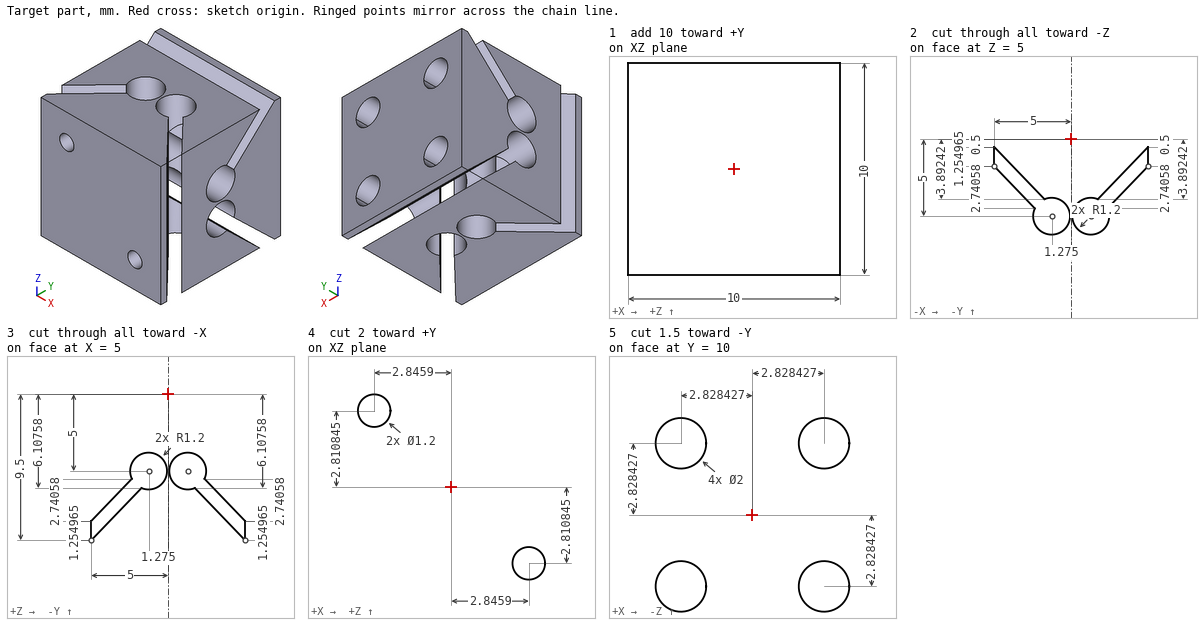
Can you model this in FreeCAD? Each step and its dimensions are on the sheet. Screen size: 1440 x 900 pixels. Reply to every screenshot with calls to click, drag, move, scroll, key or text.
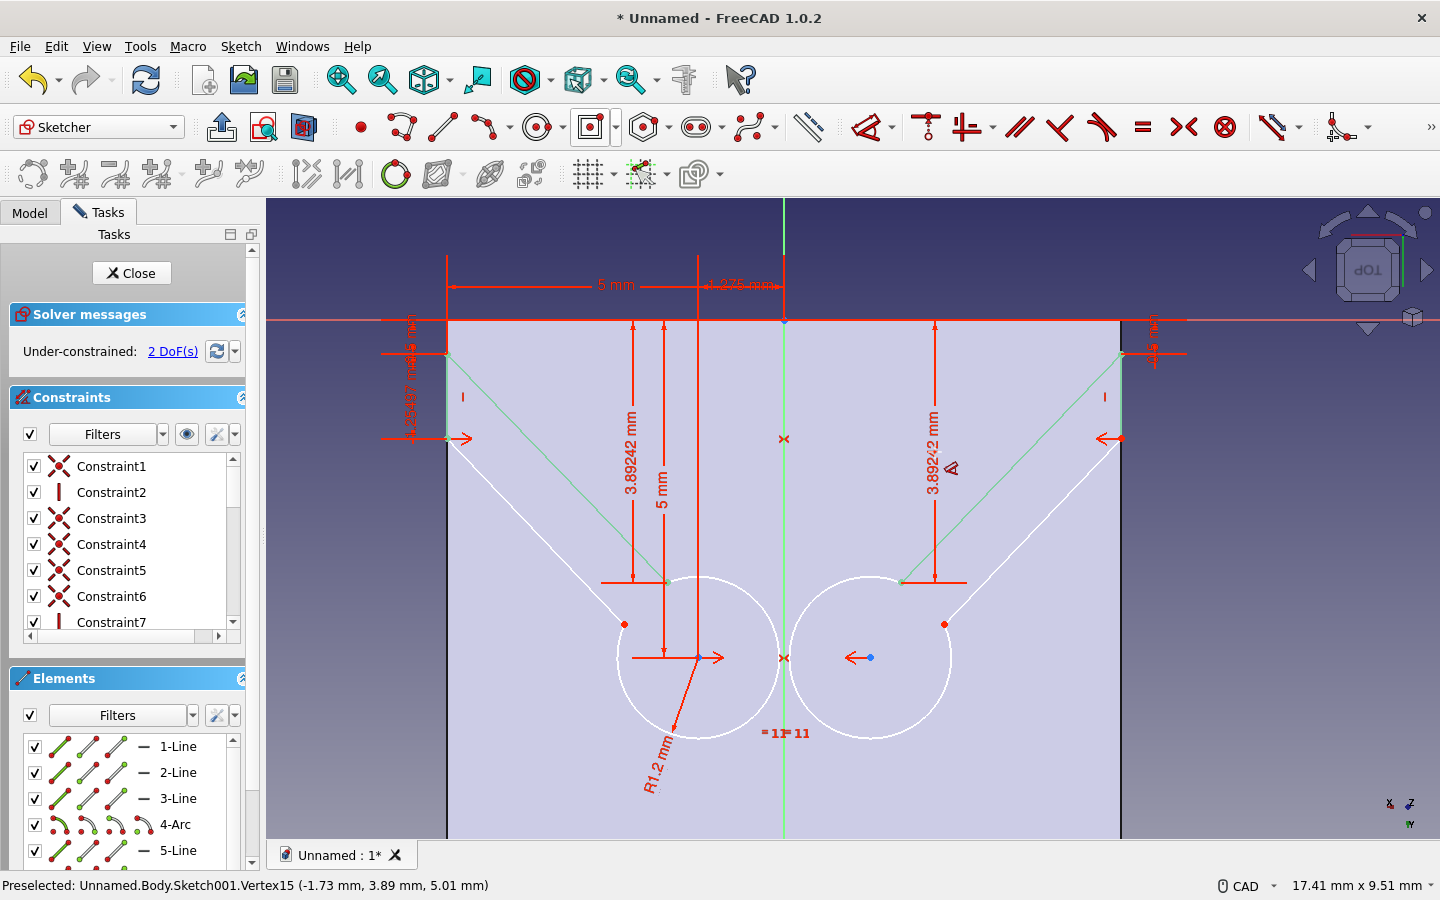
click(500, 495)
click(413, 532)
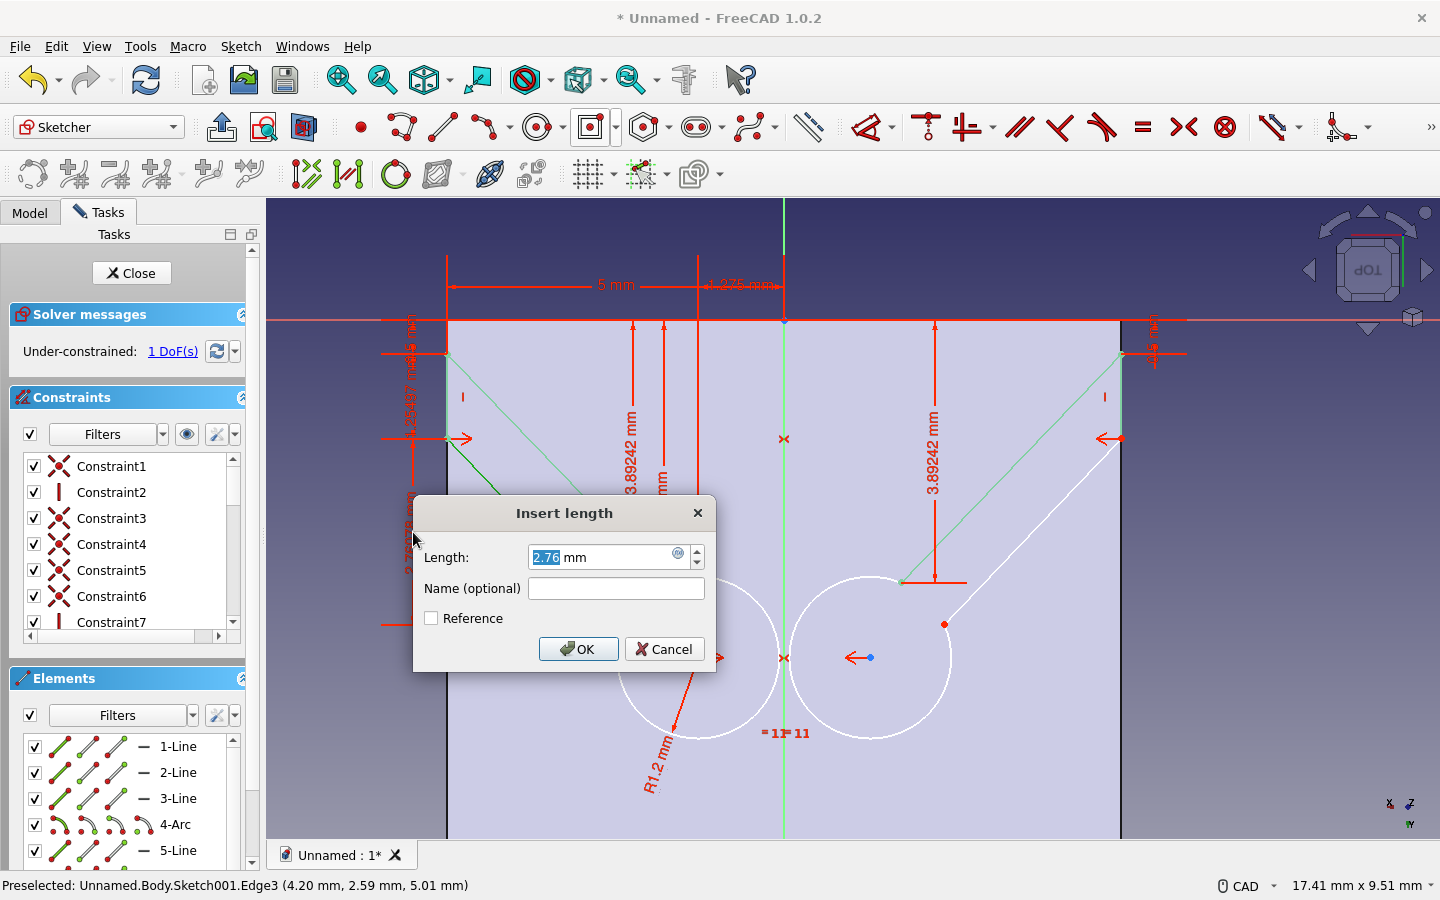
text(2.74058)
key(Return)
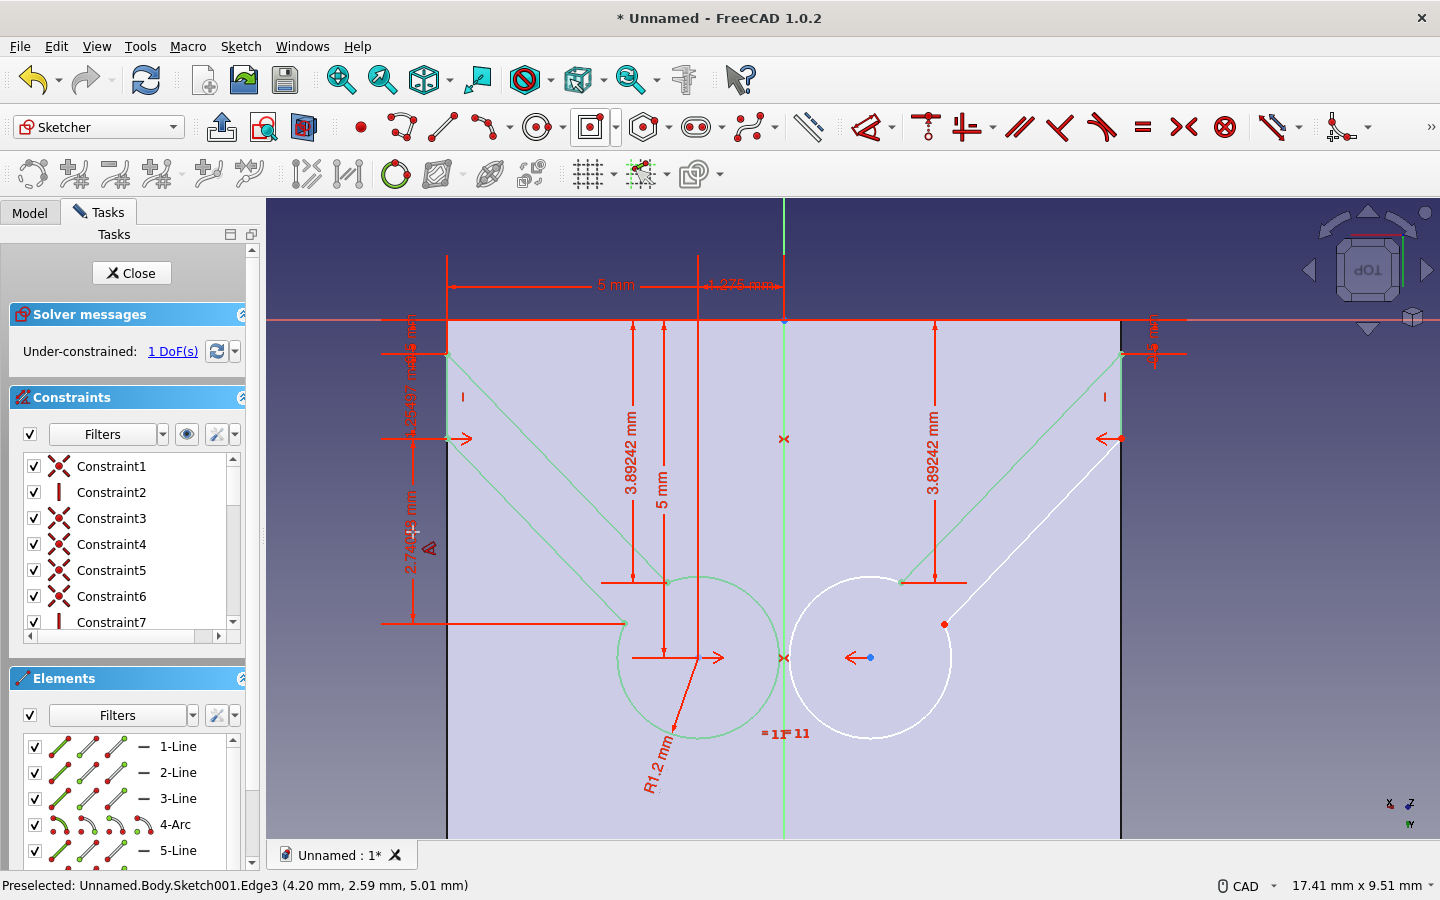
click(997, 569)
click(1155, 532)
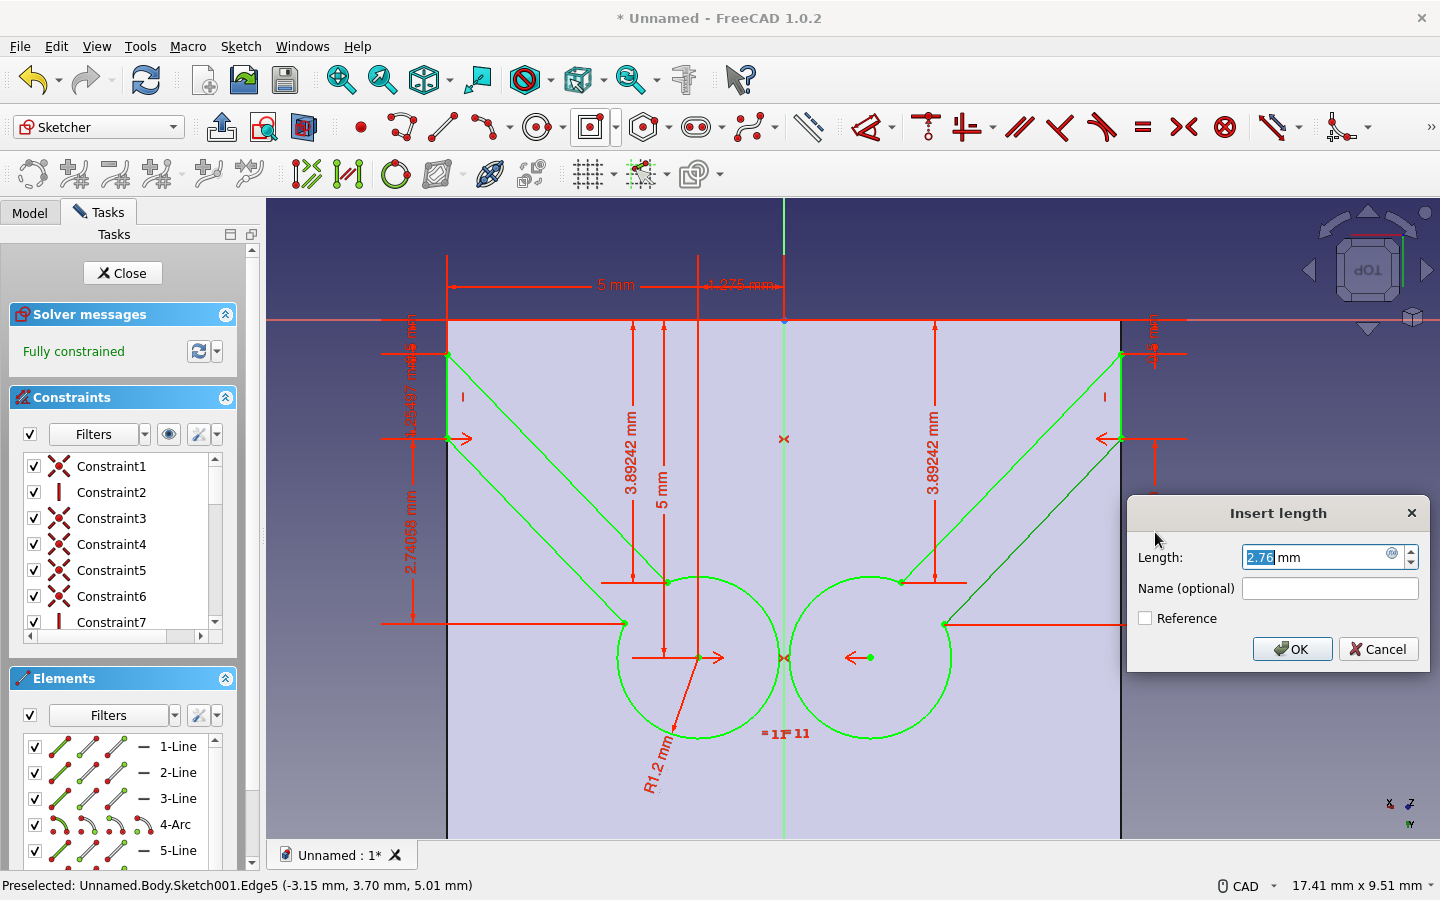
text(2.74058)
key(Return)
key(Escape)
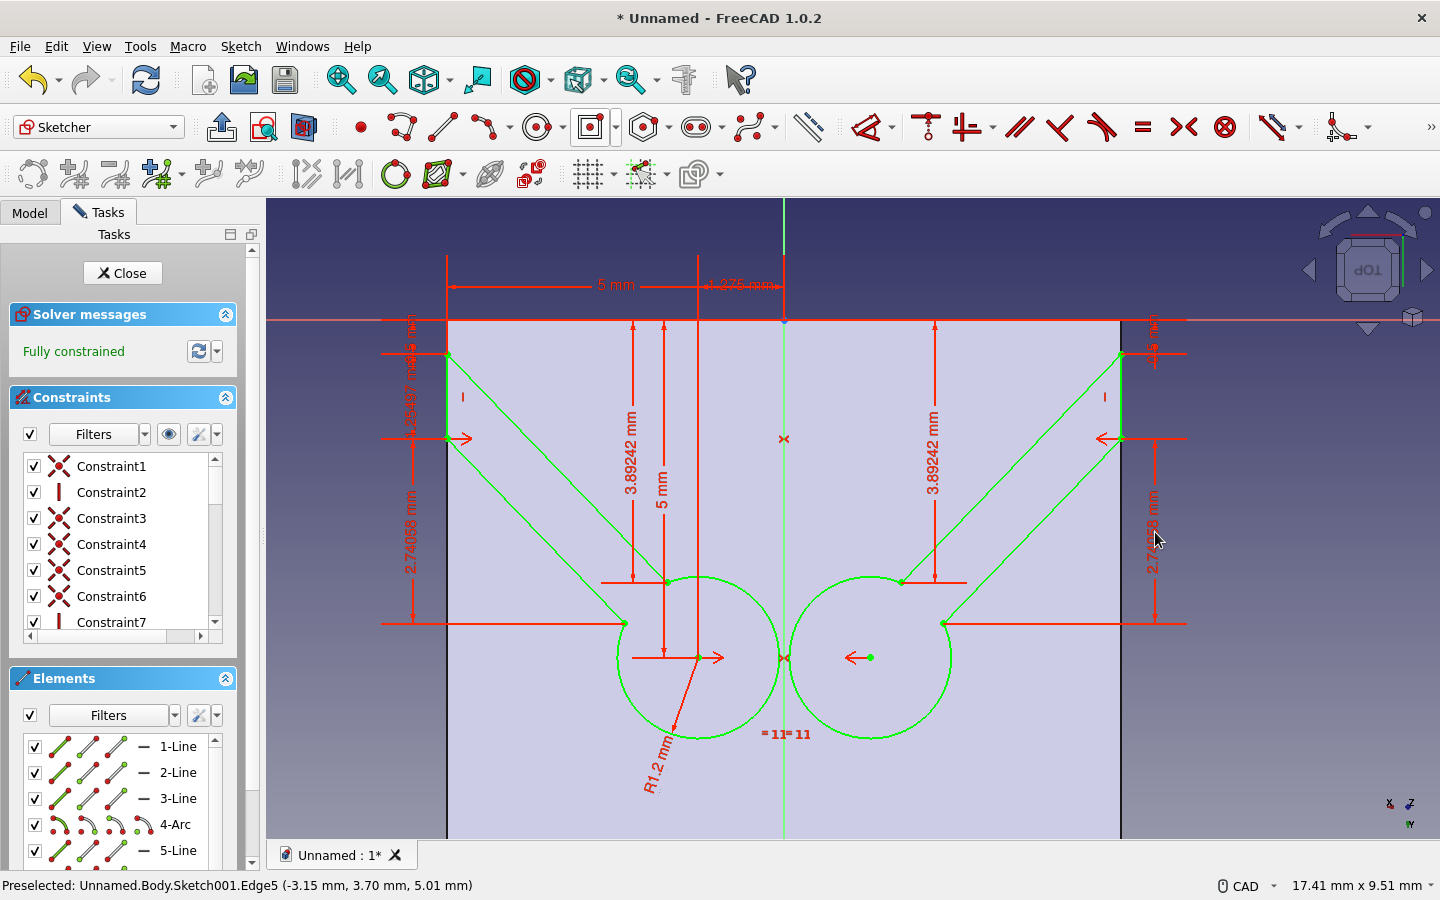
click(123, 273)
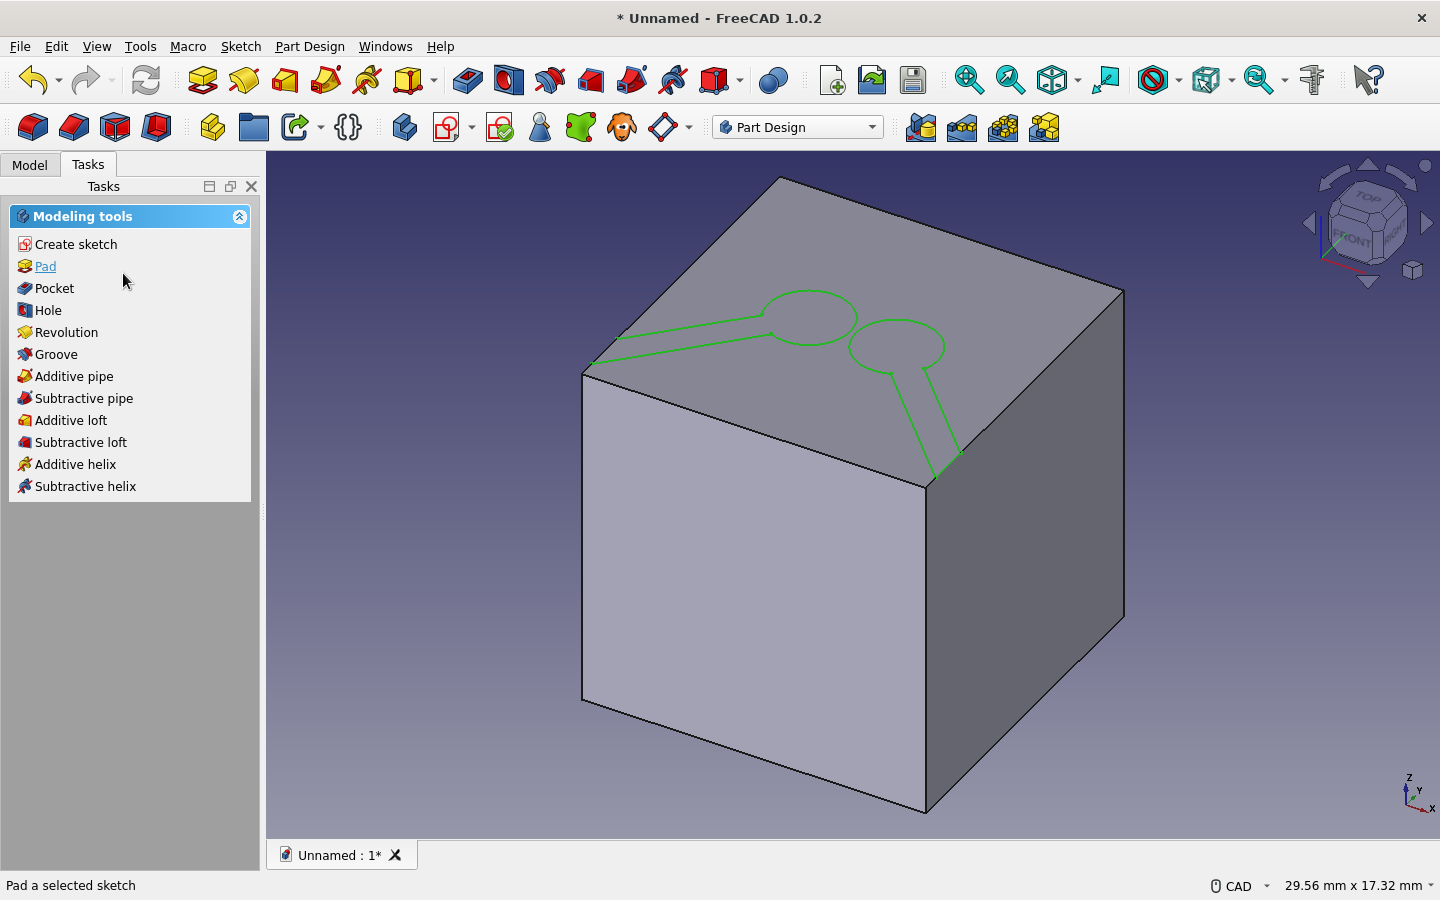
click(468, 80)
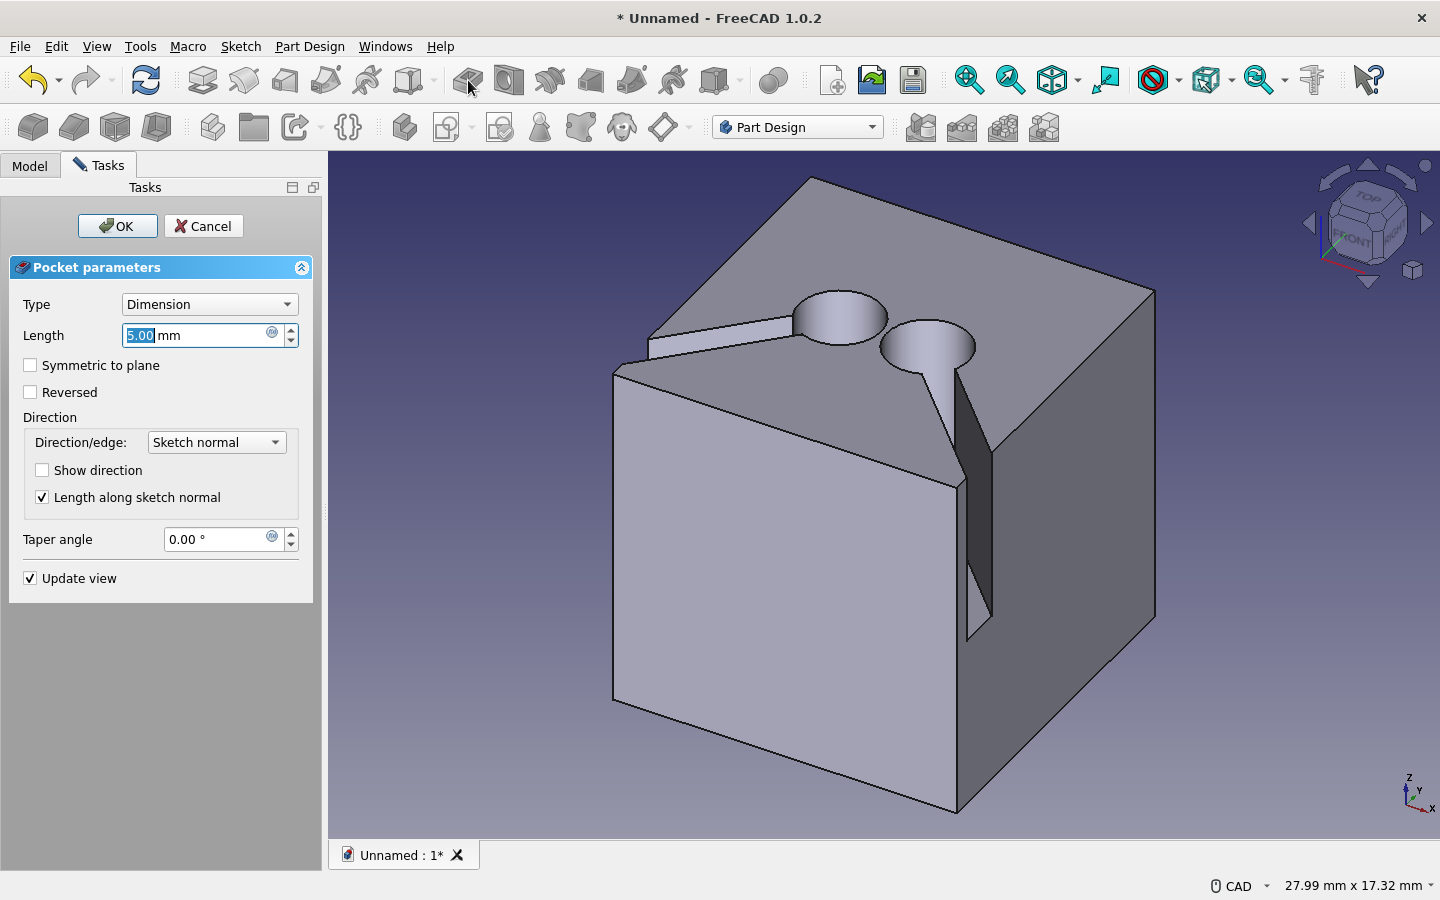
click(210, 304)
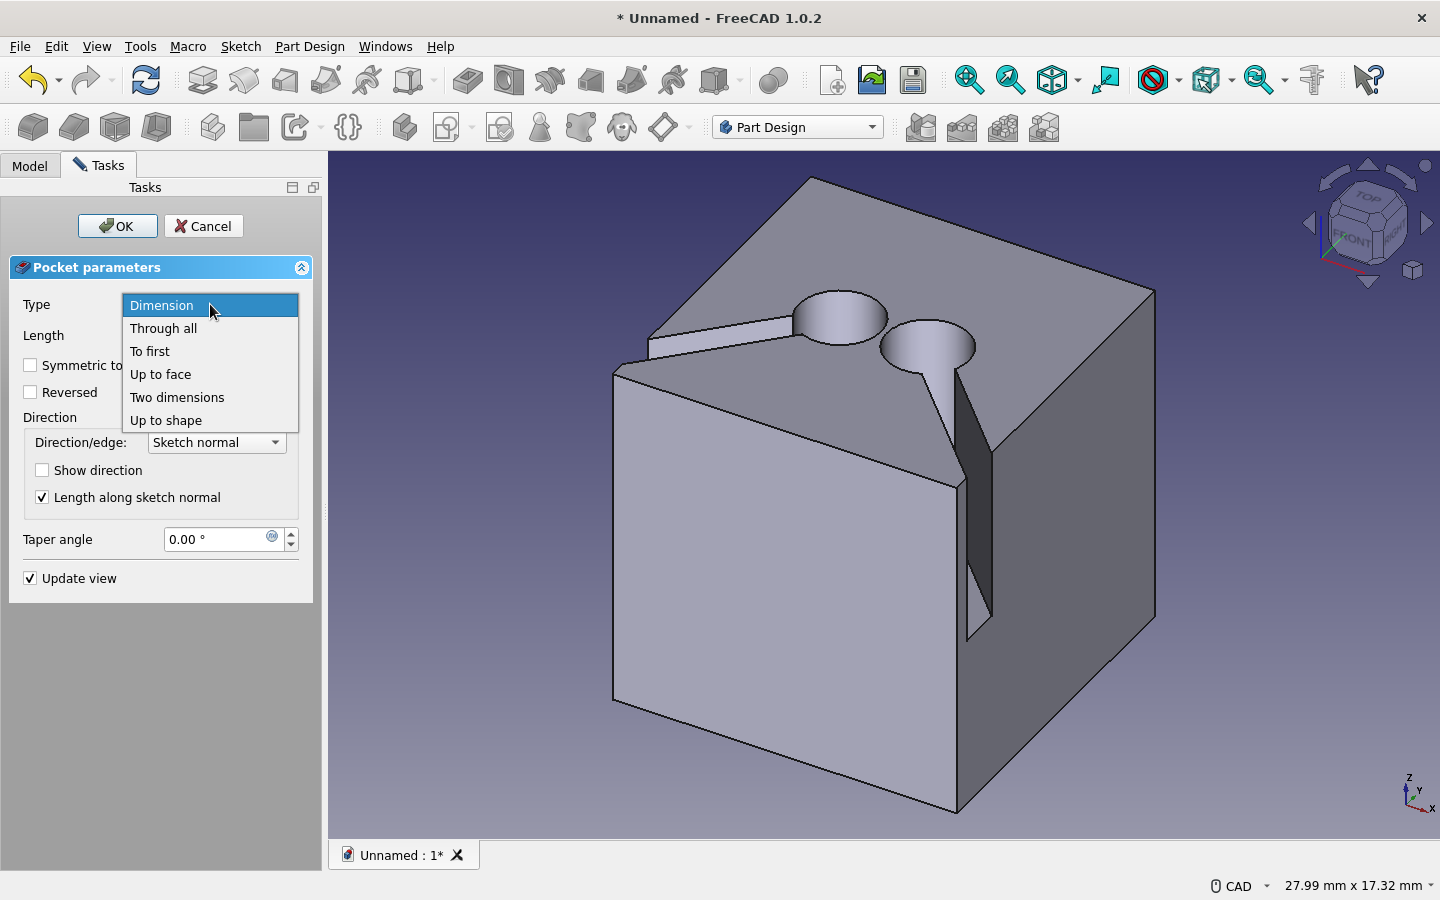
click(208, 328)